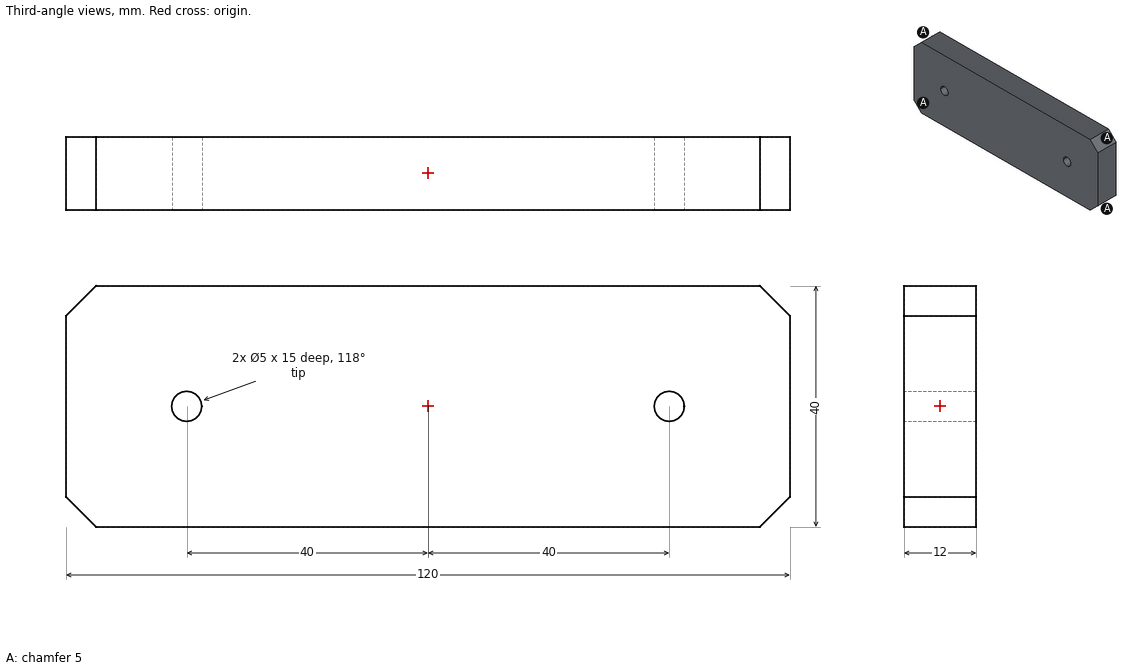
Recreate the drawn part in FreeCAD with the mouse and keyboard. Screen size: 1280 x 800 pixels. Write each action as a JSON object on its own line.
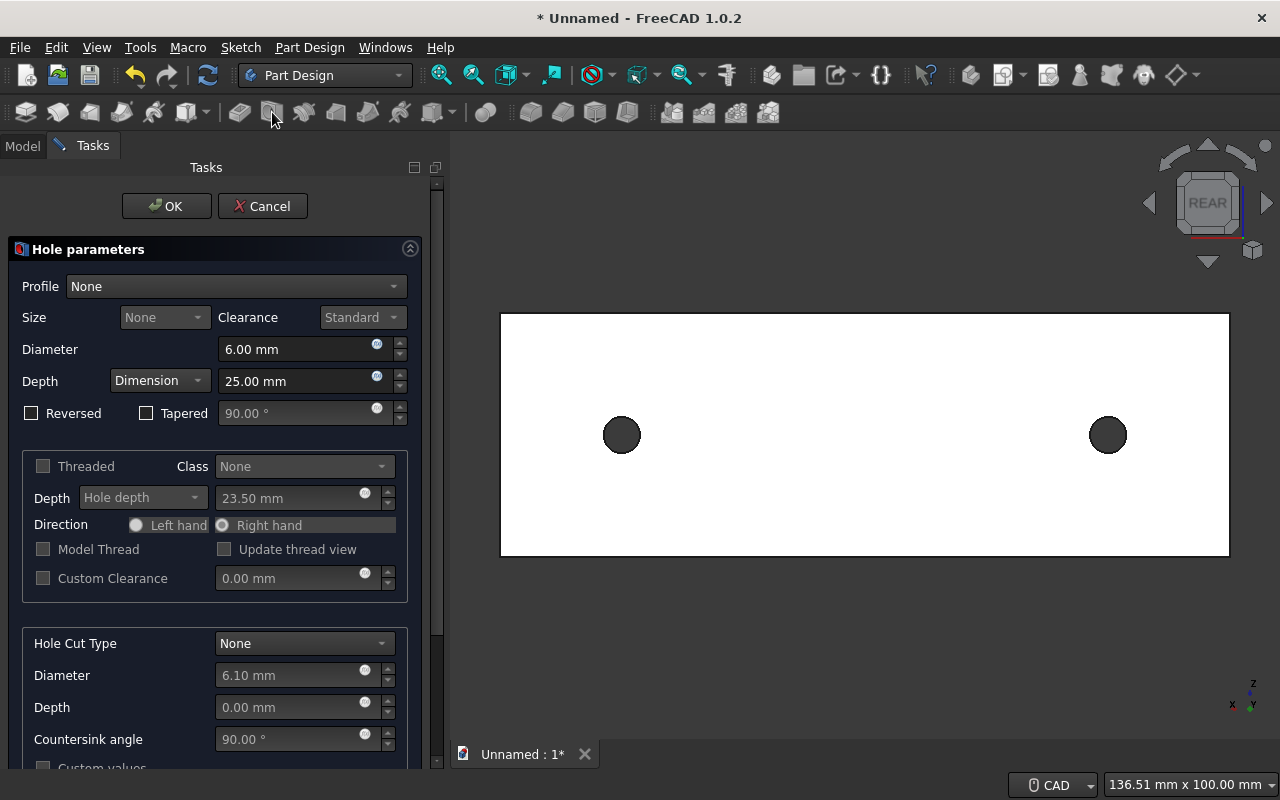
{"action": "triple_click", "coordinate": [305, 349]}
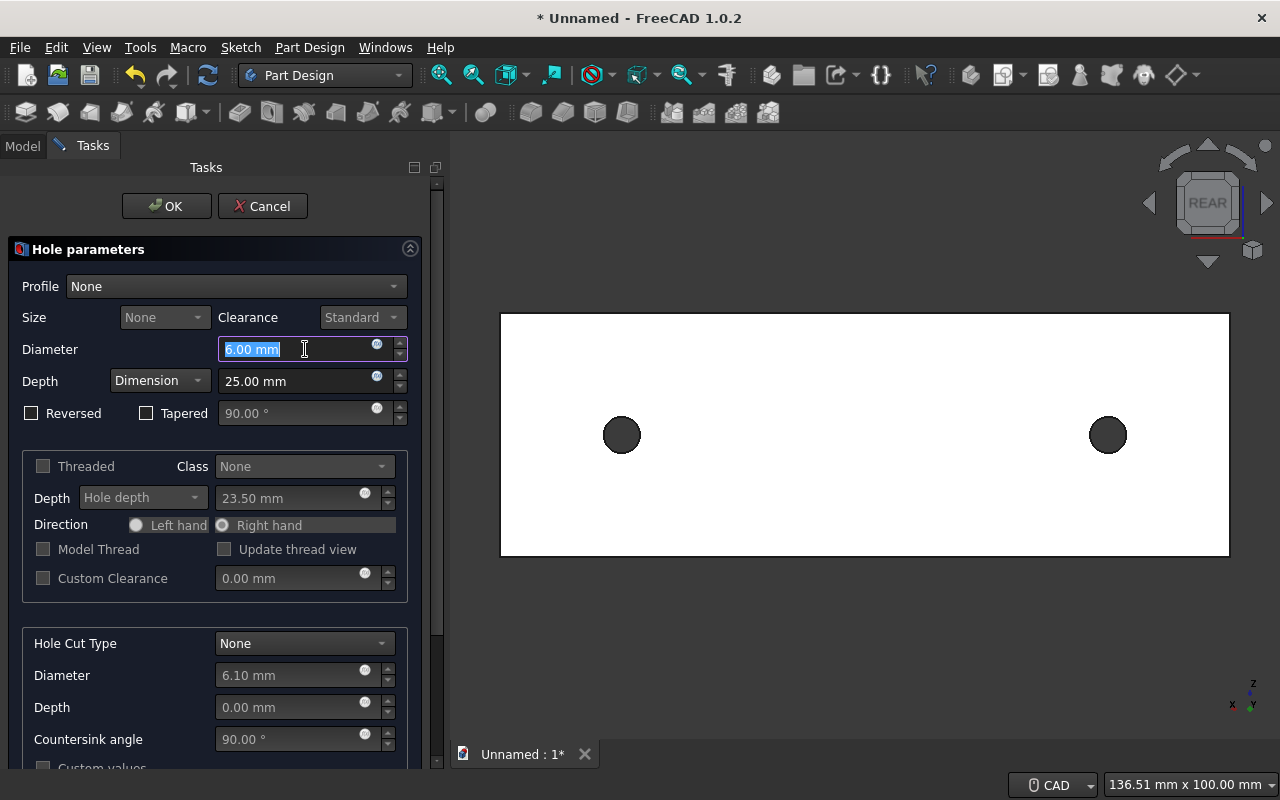
{"action": "type", "text": "5"}
{"action": "key", "text": "Tab"}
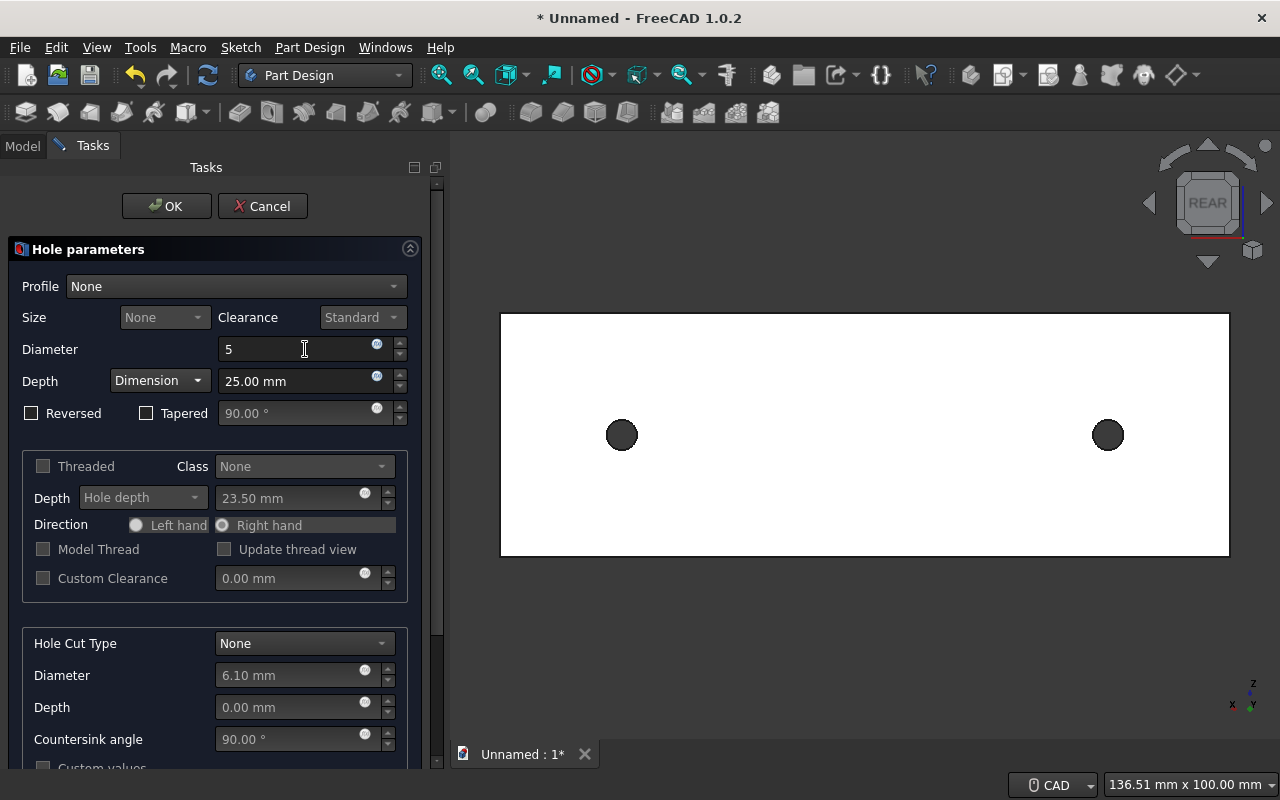
{"action": "triple_click", "coordinate": [305, 381]}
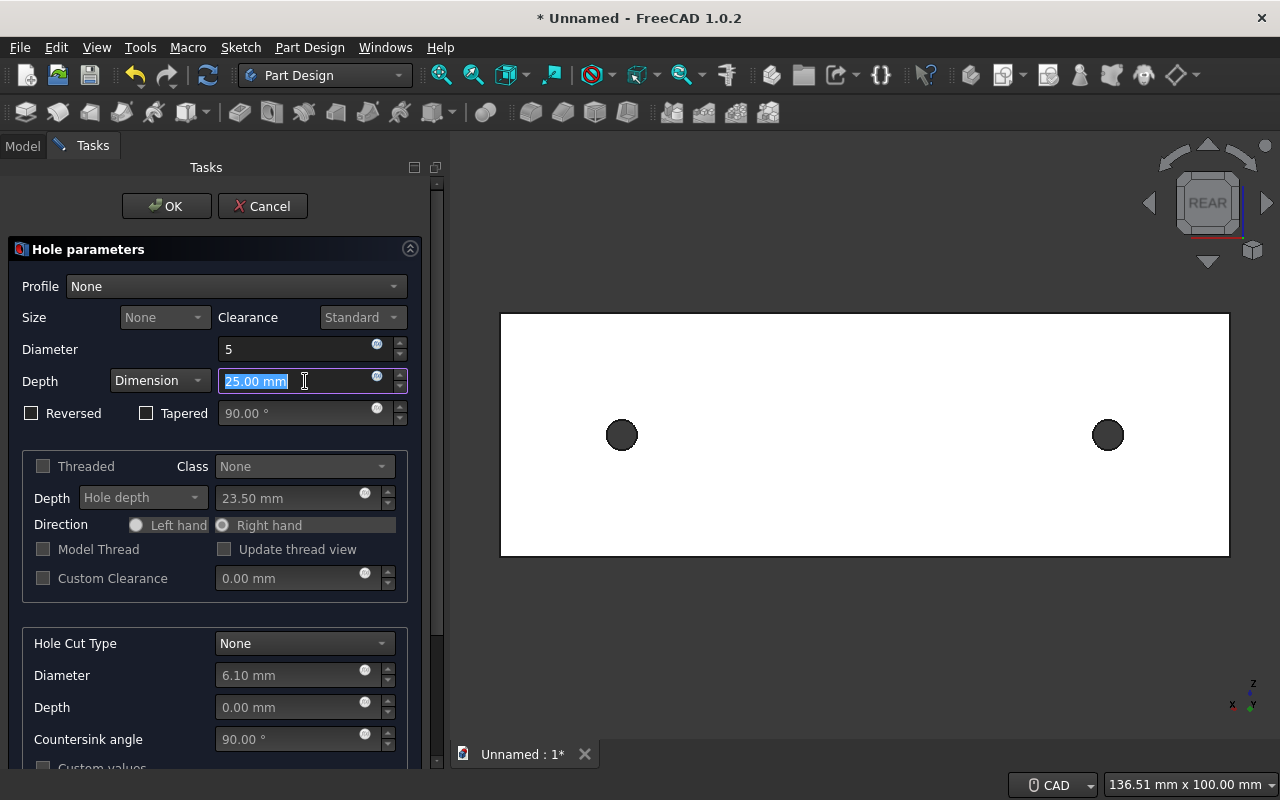
{"action": "type", "text": "15"}
{"action": "key", "text": "Tab"}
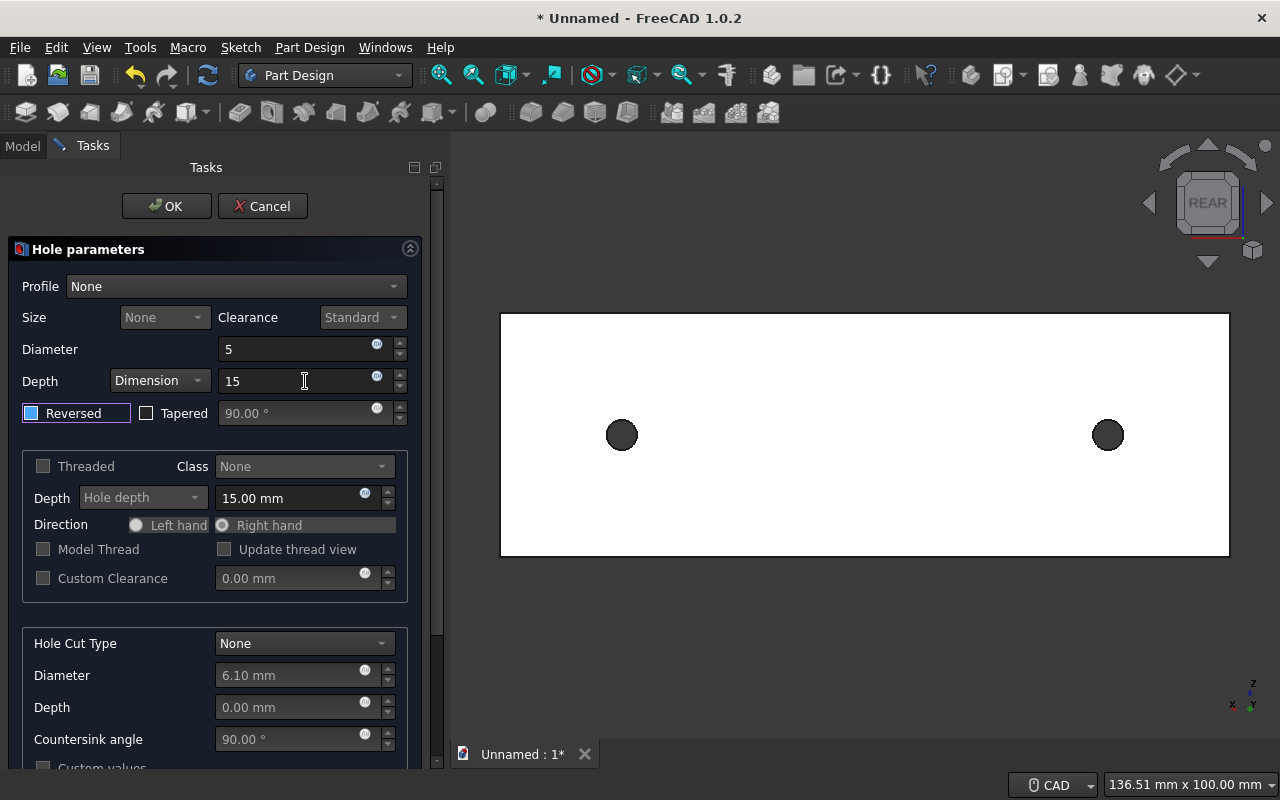
{"action": "left_click", "coordinate": [167, 206]}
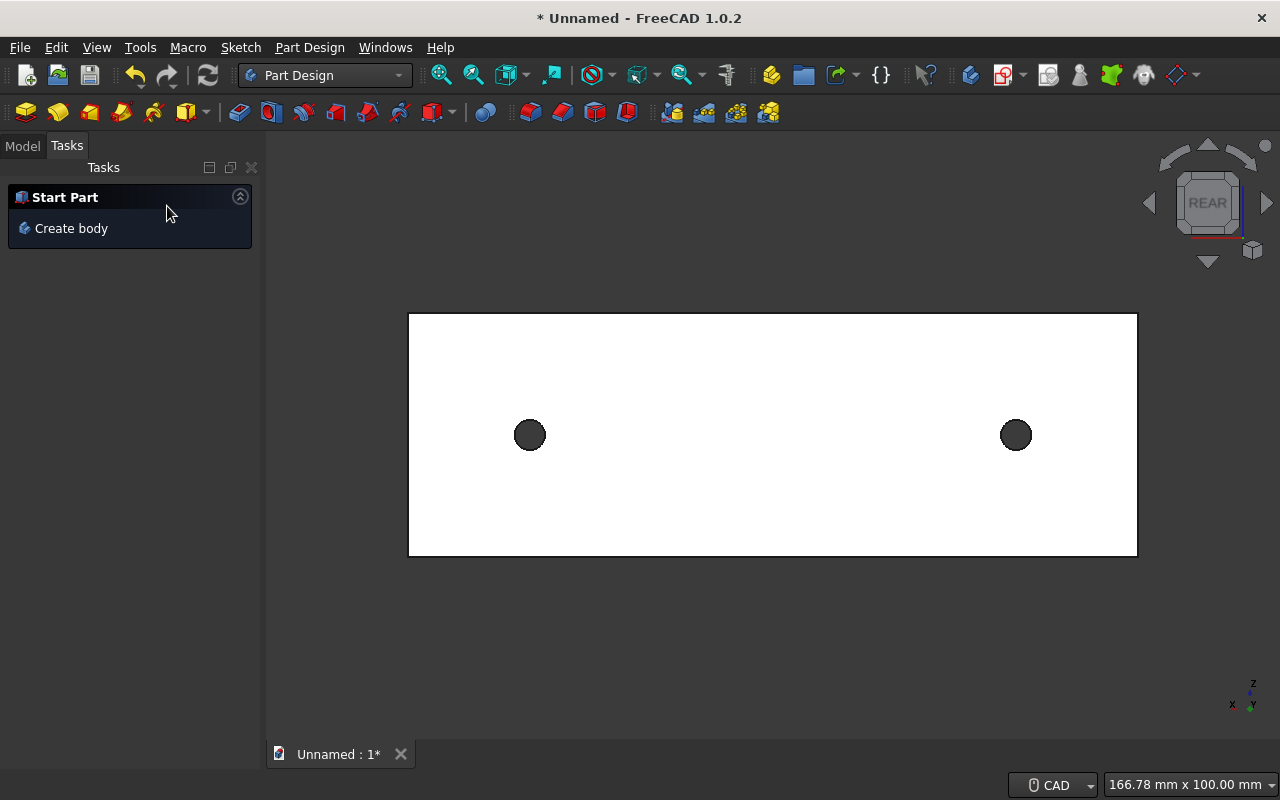
{"action": "key", "text": "0"}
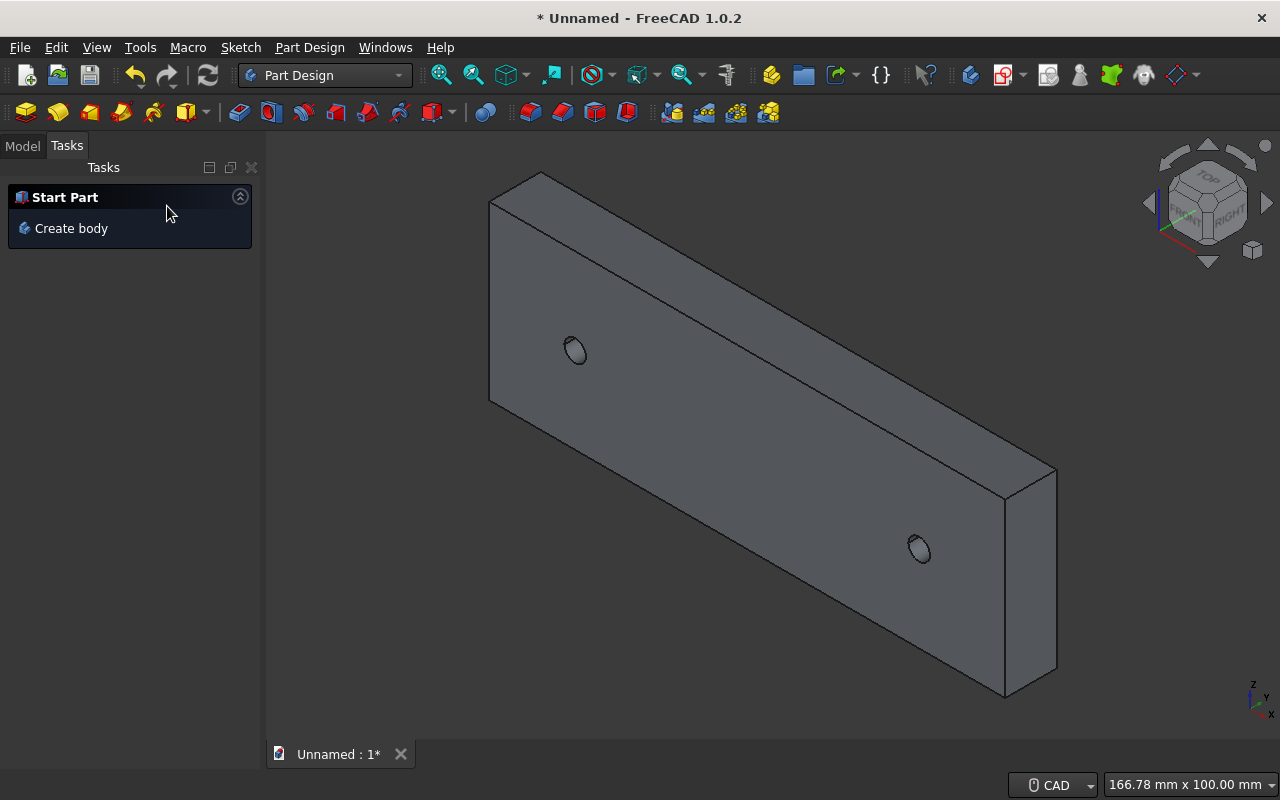
{"action": "left_click", "coordinate": [1031, 484]}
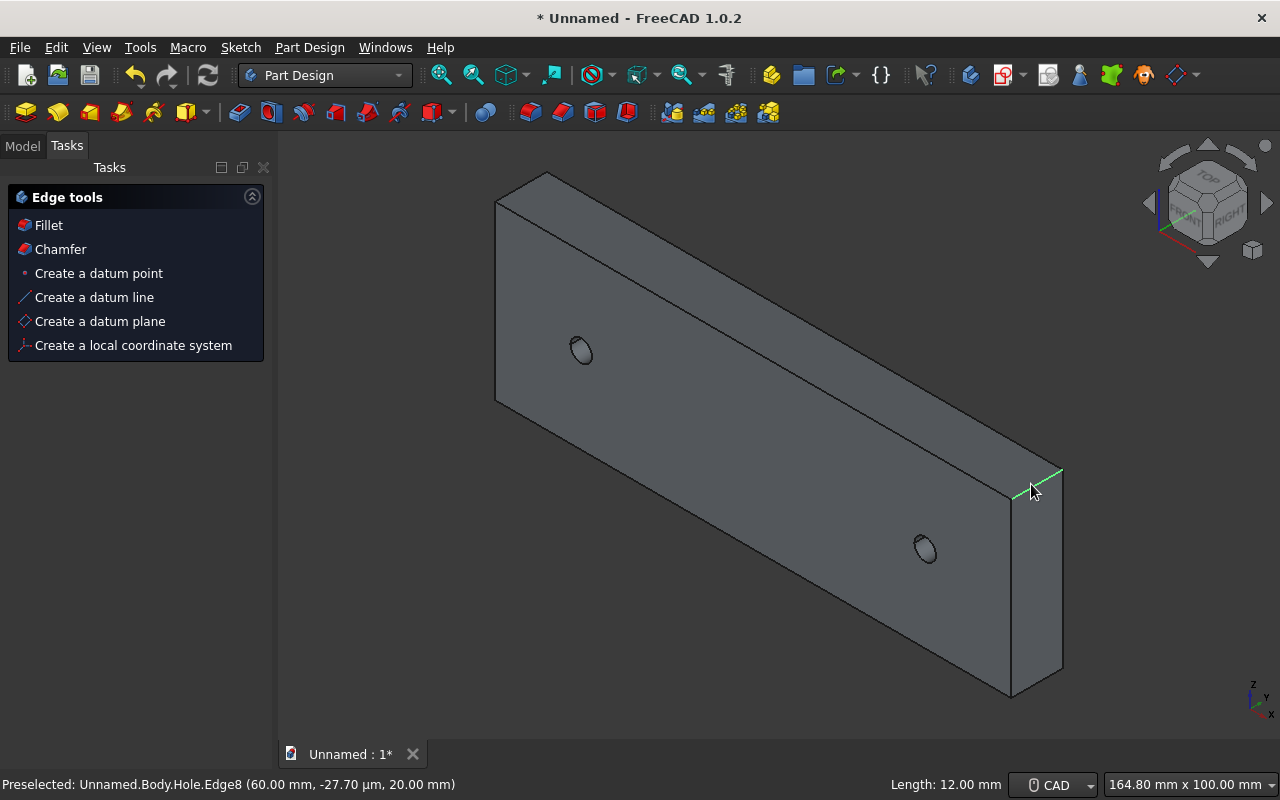
{"action": "key", "text": "2"}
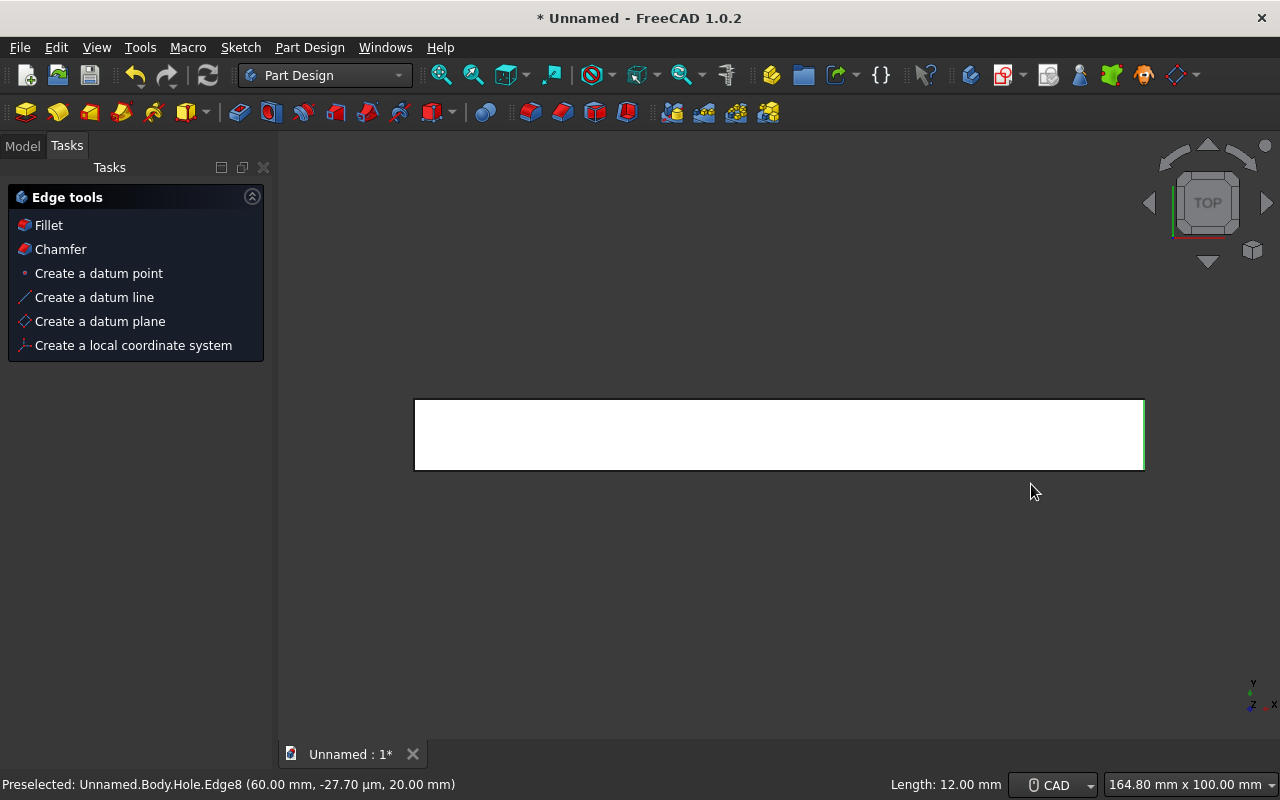
{"action": "left_click", "coordinate": [414, 434], "text": "ctrl"}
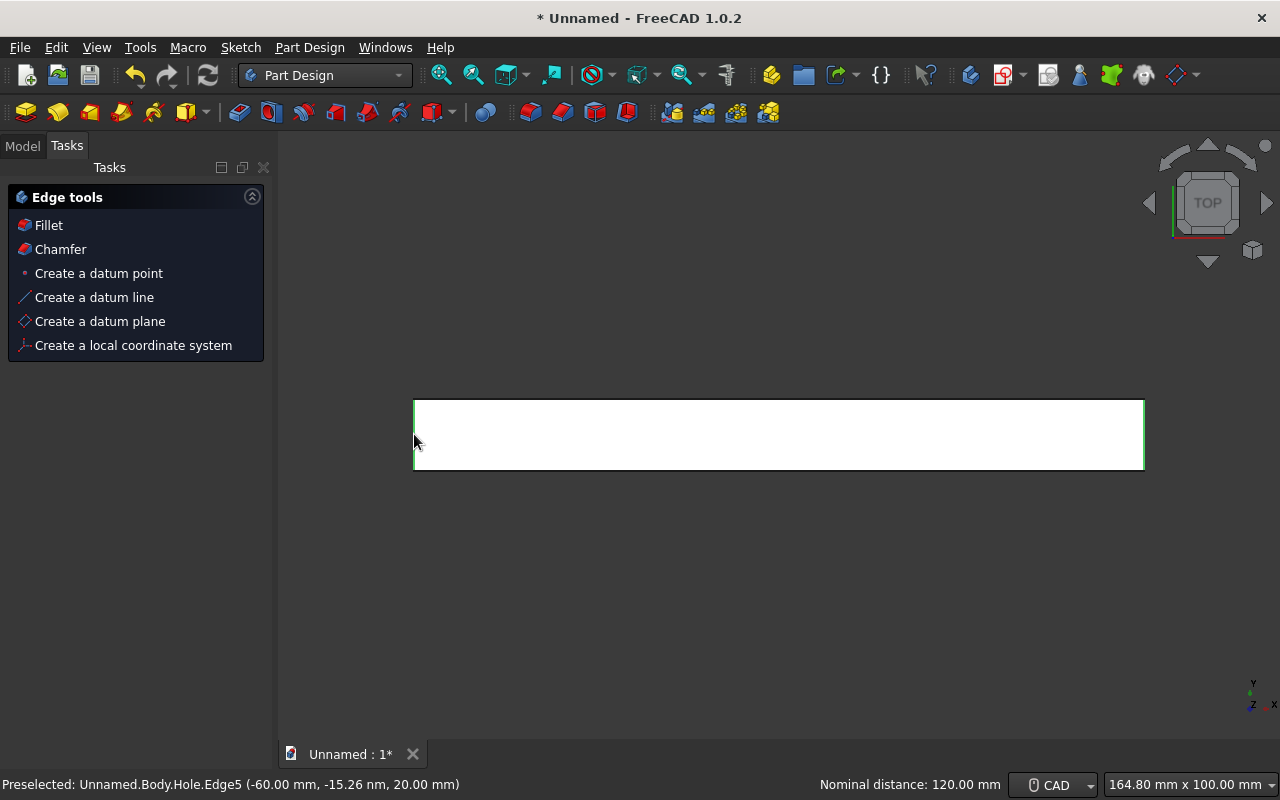
{"action": "key", "text": "1"}